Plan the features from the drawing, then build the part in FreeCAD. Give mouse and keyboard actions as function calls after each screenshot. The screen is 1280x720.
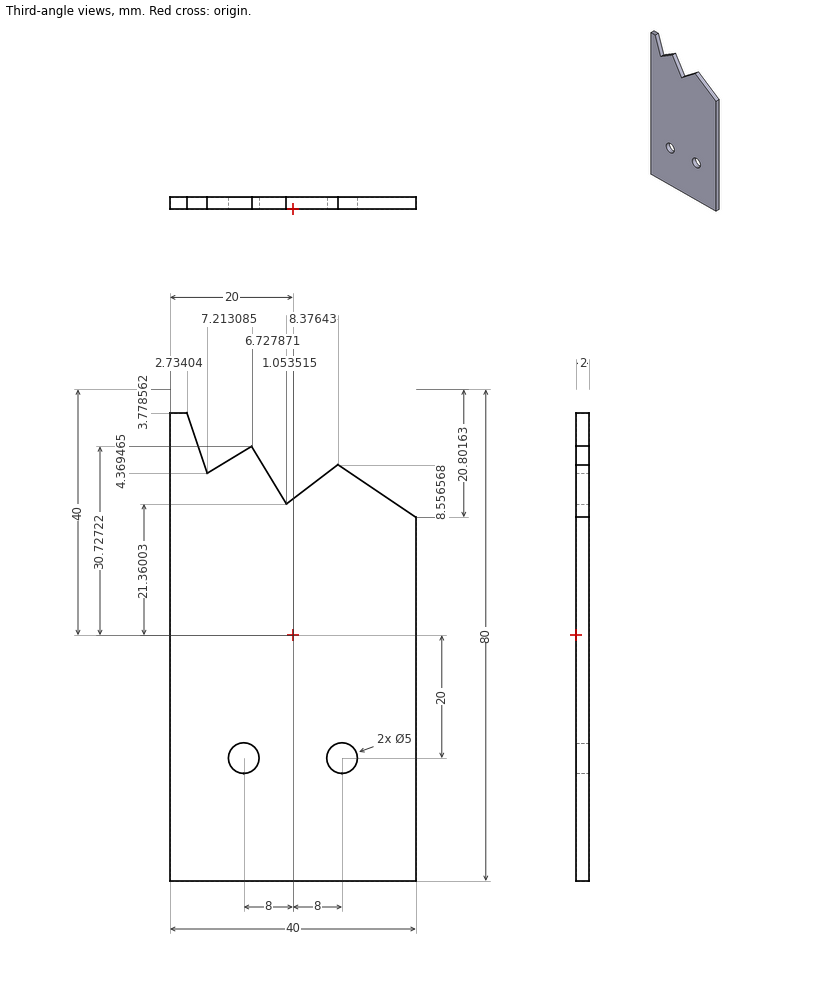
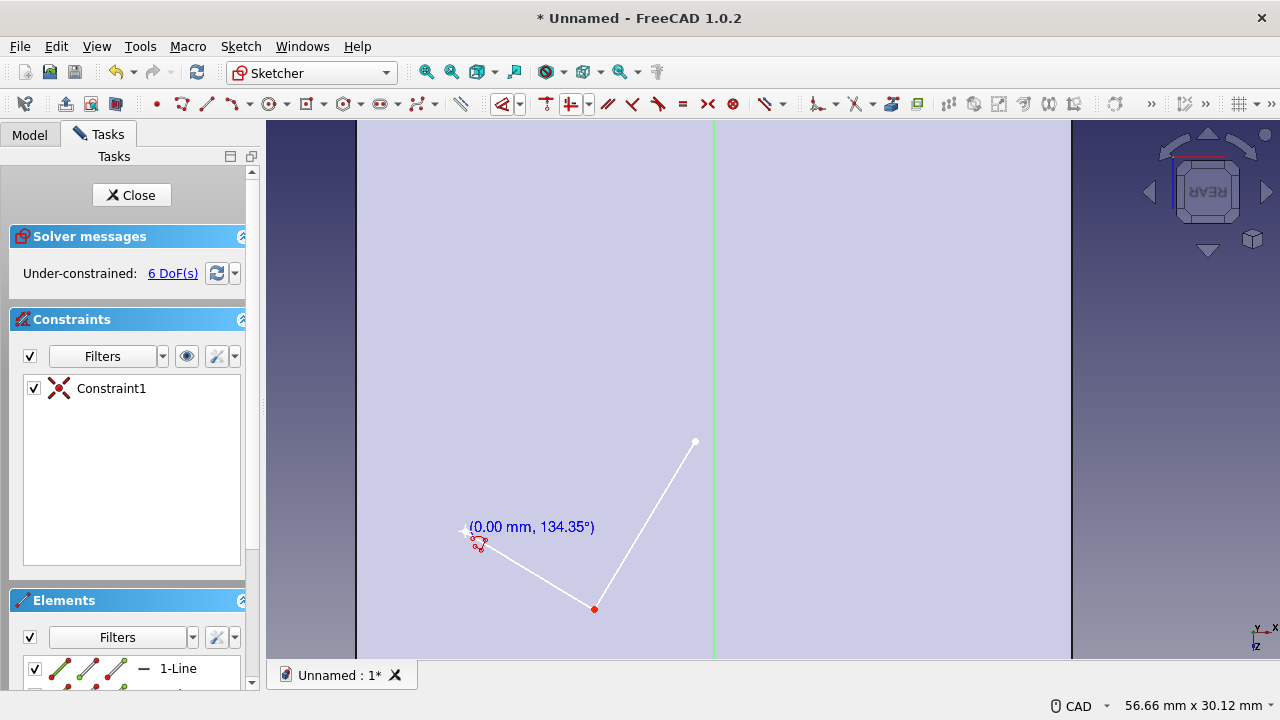
scroll(697, 367, down, 4)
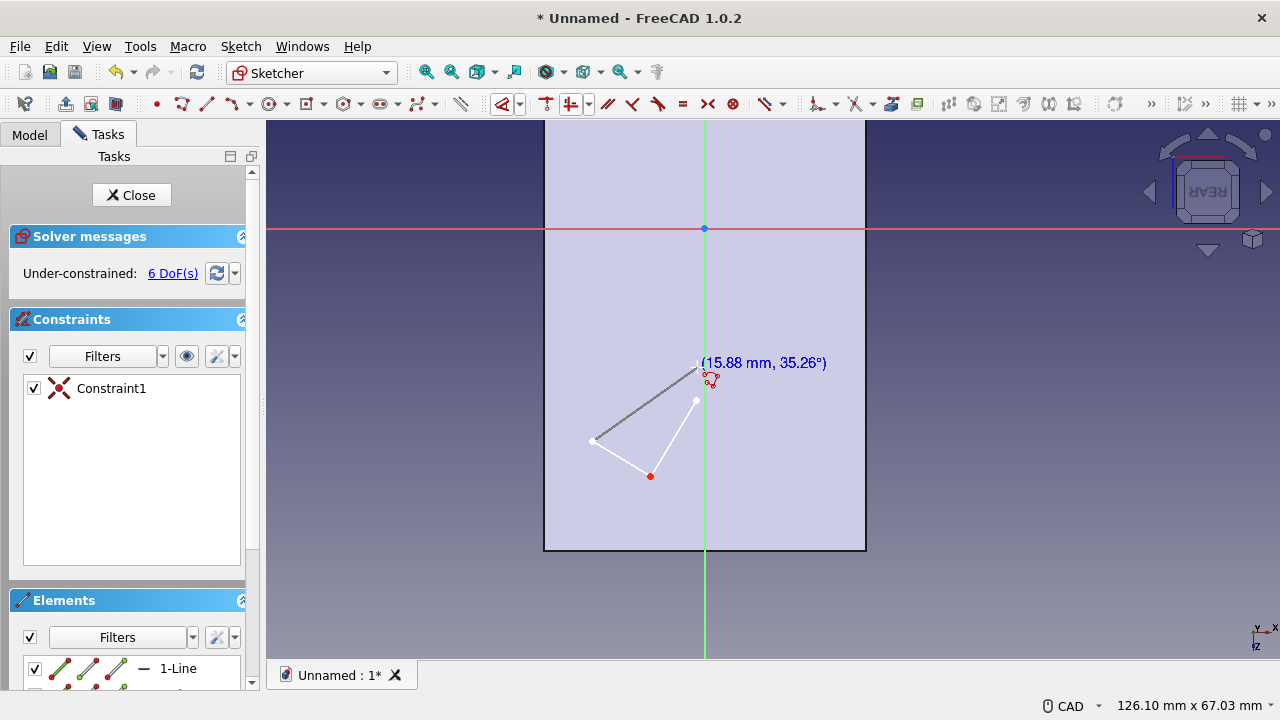
click(566, 520)
click(544, 520)
click(544, 551)
click(866, 551)
click(866, 383)
click(764, 452)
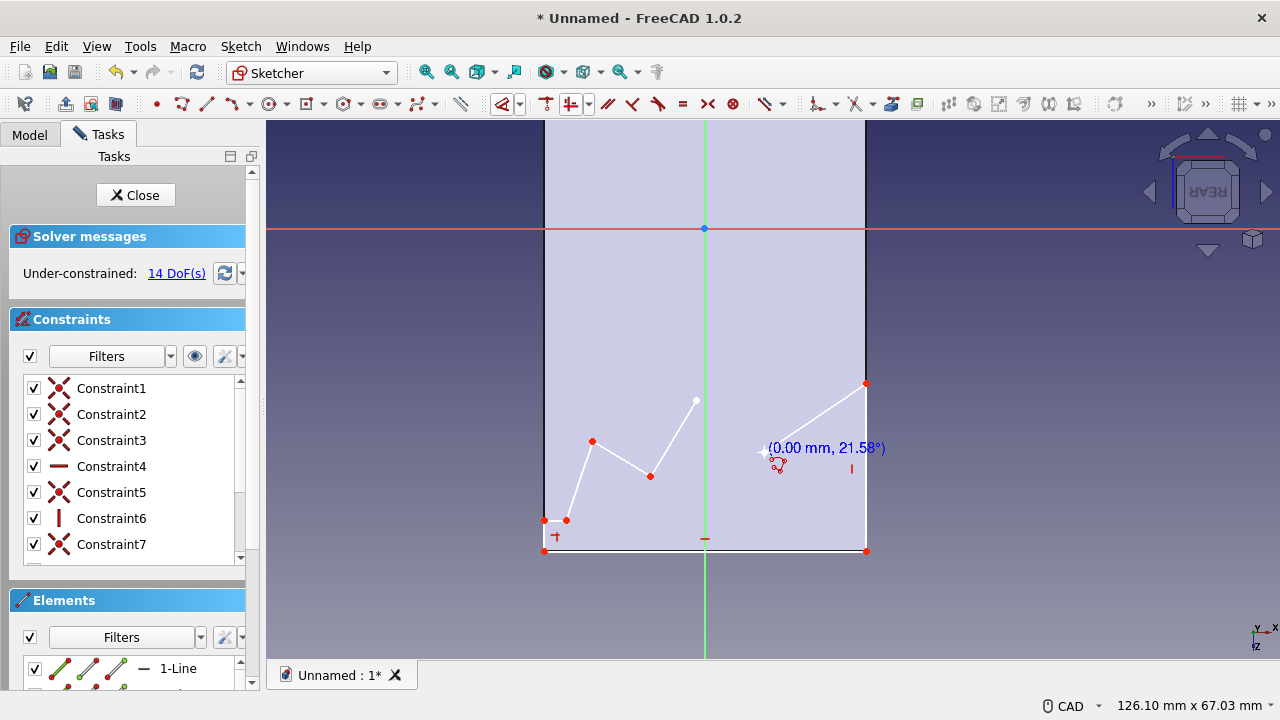
scroll(696, 401, up, 4)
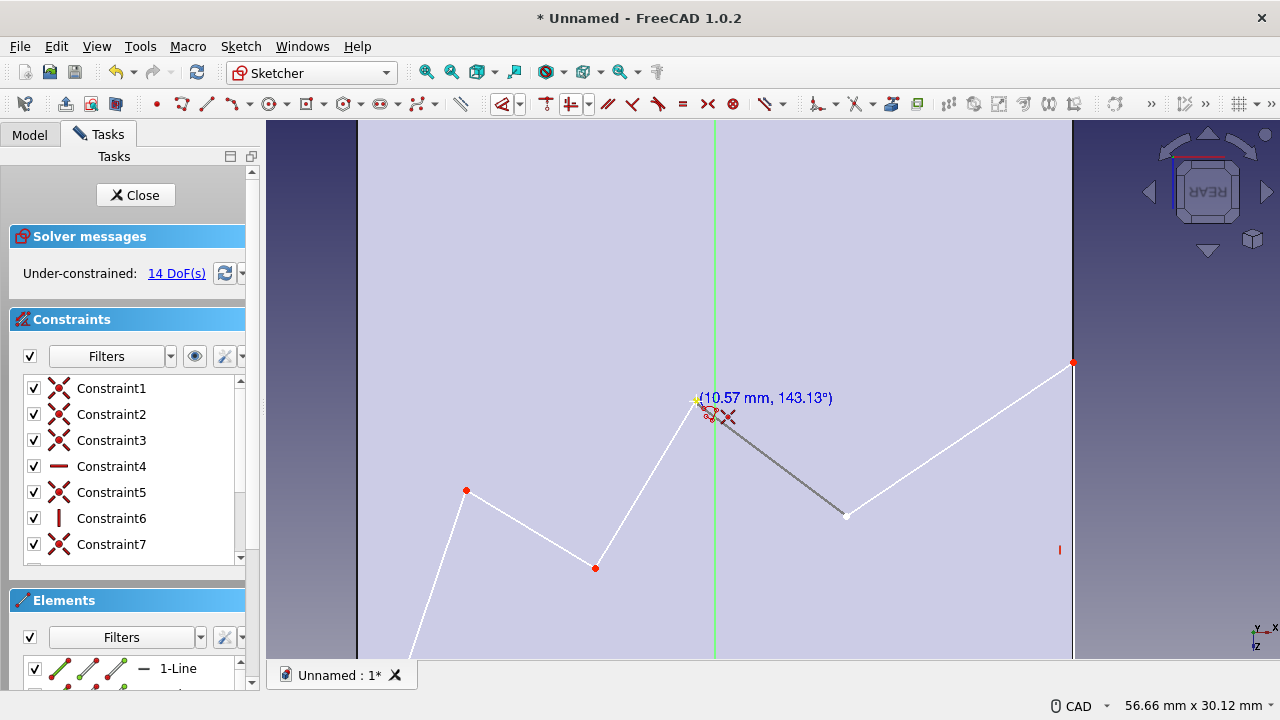
click(696, 400)
key(Escape)
key(Escape)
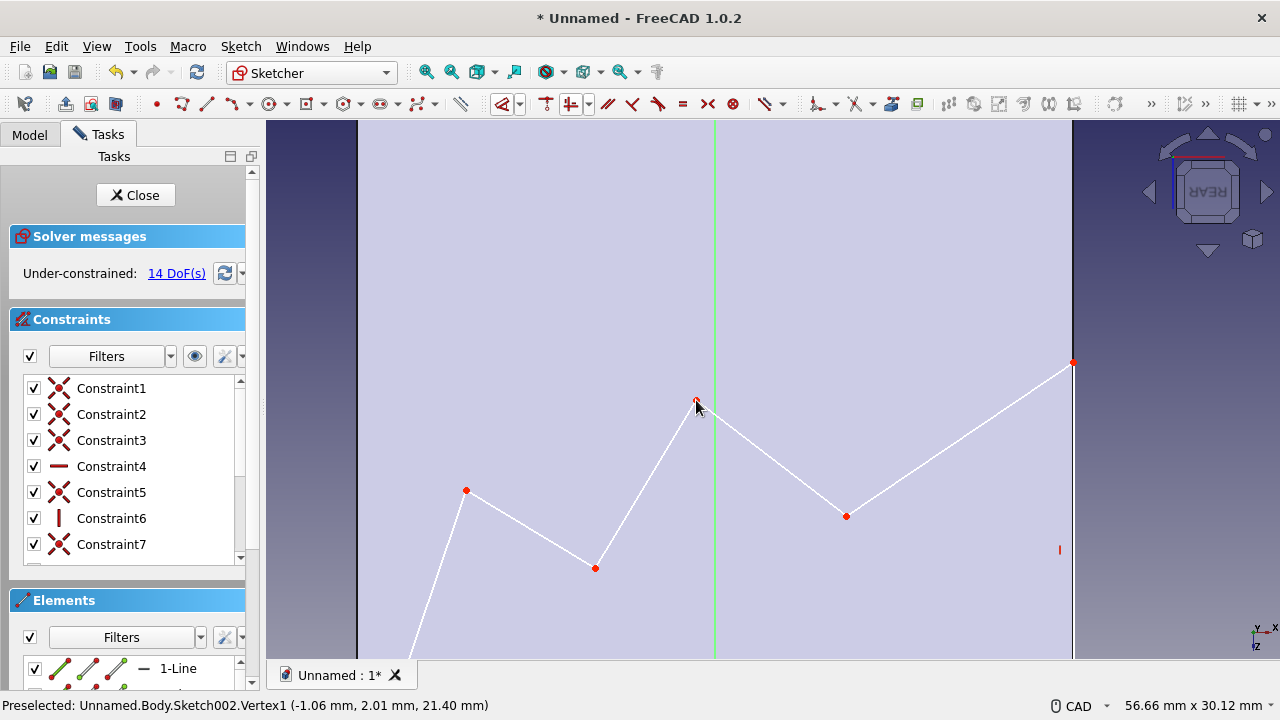
scroll(696, 401, down, 4)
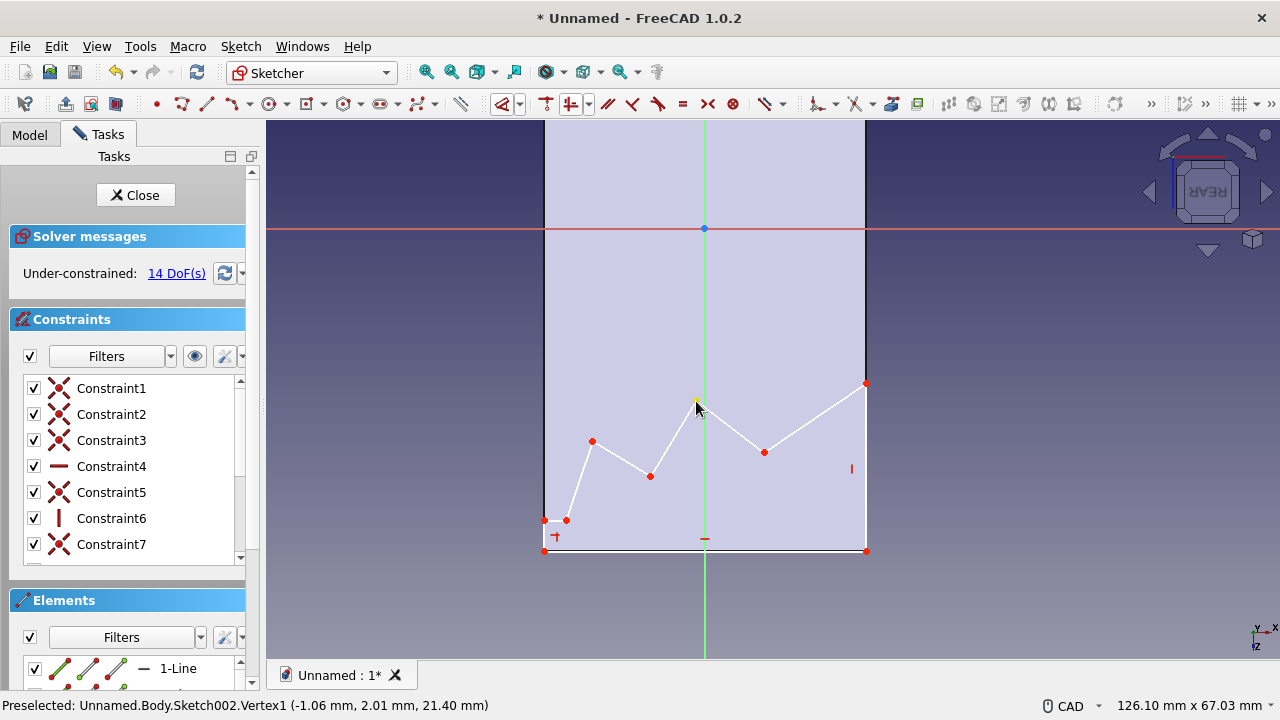
click(641, 552)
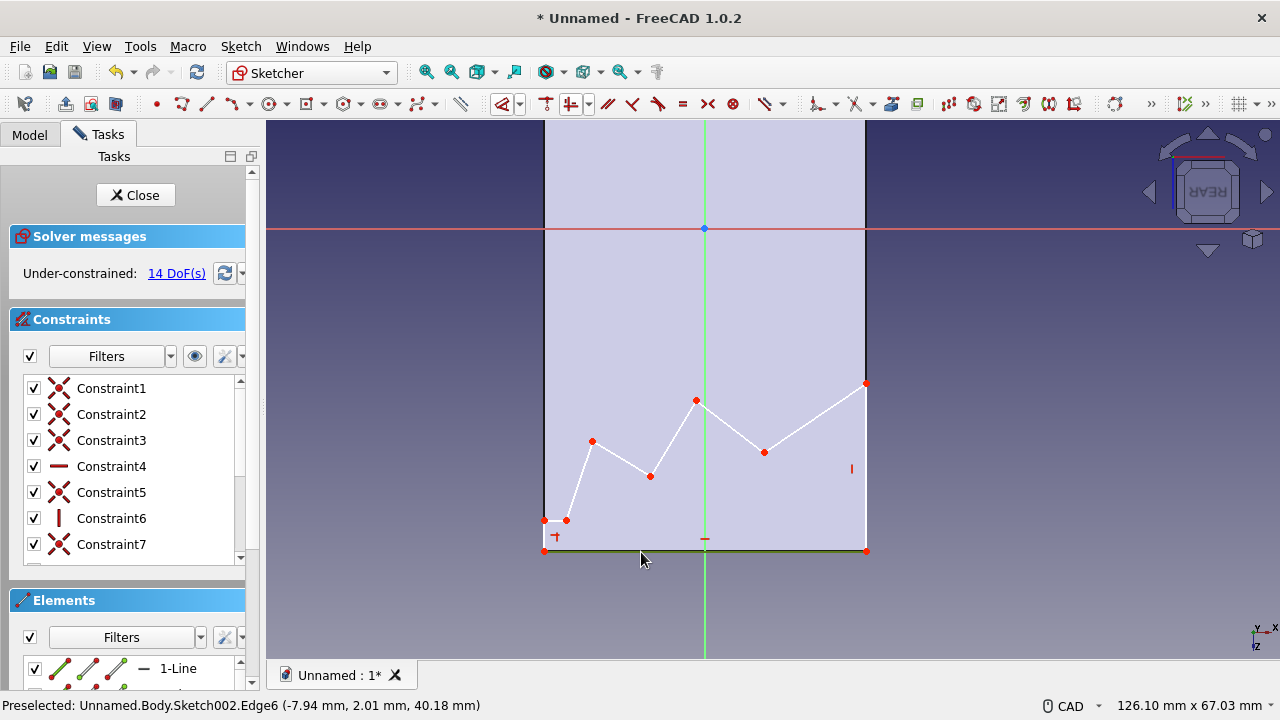
key(l)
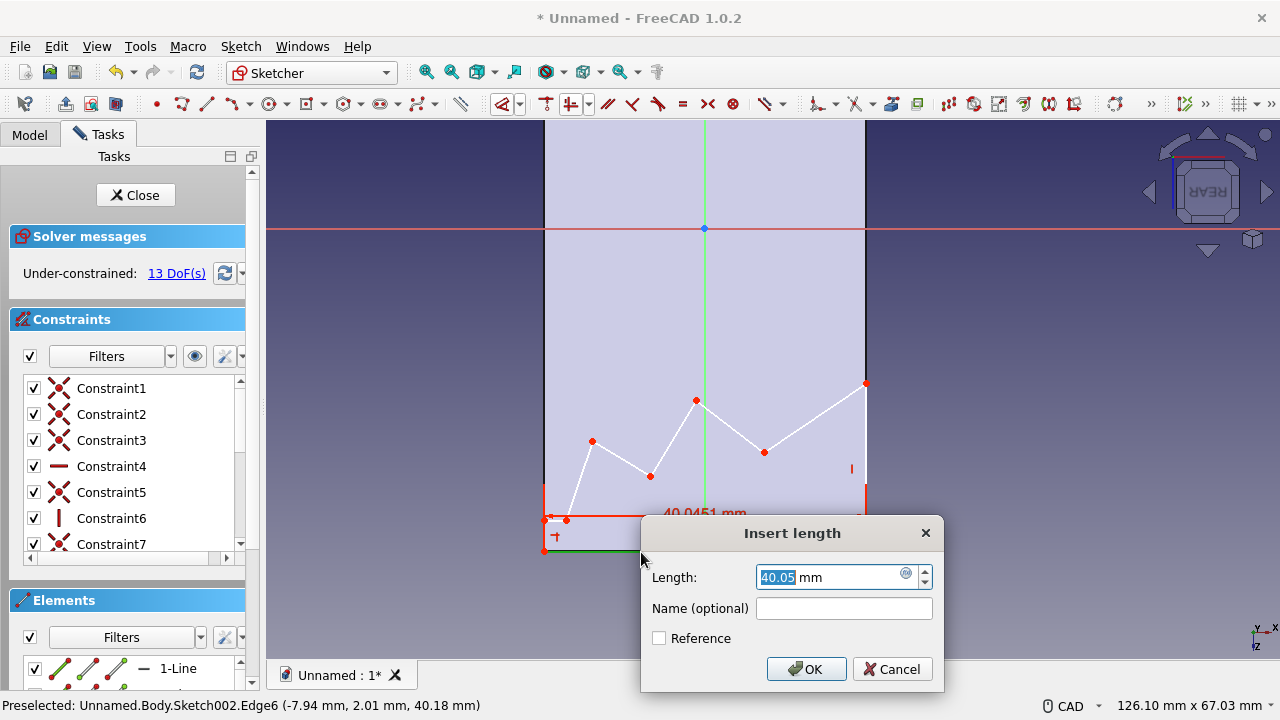
text(40)
key(Return)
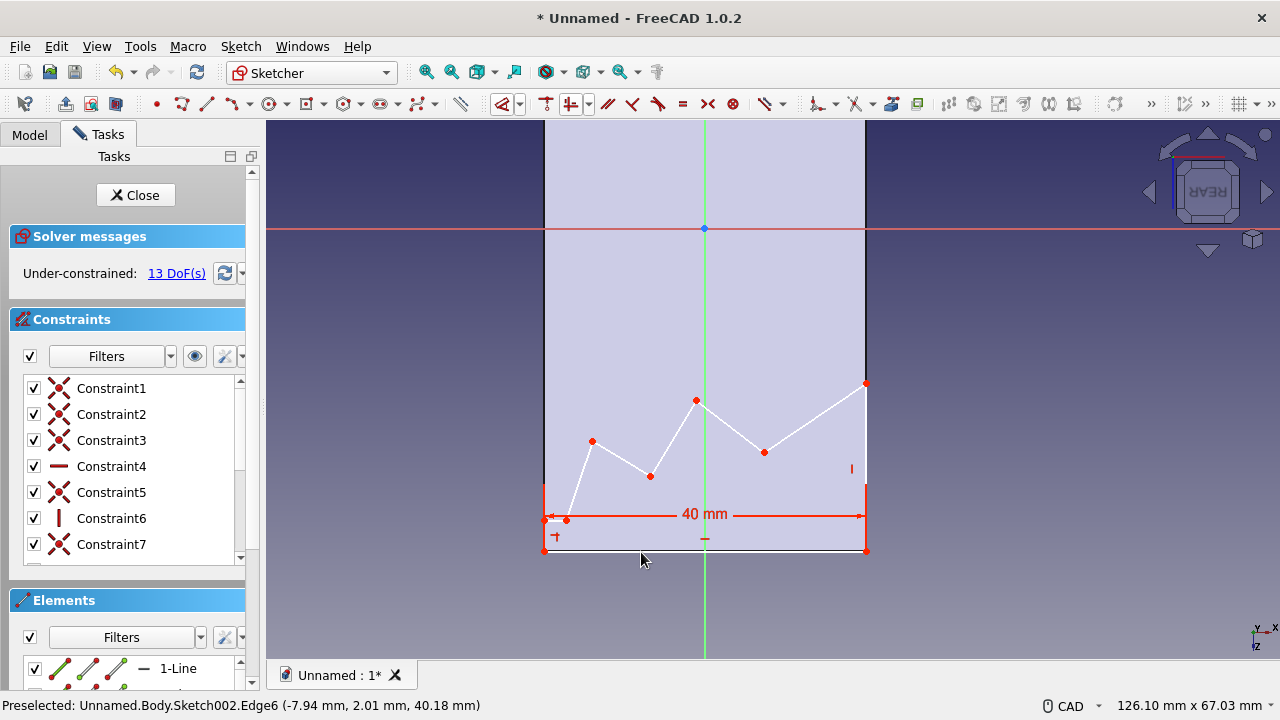
click(544, 521)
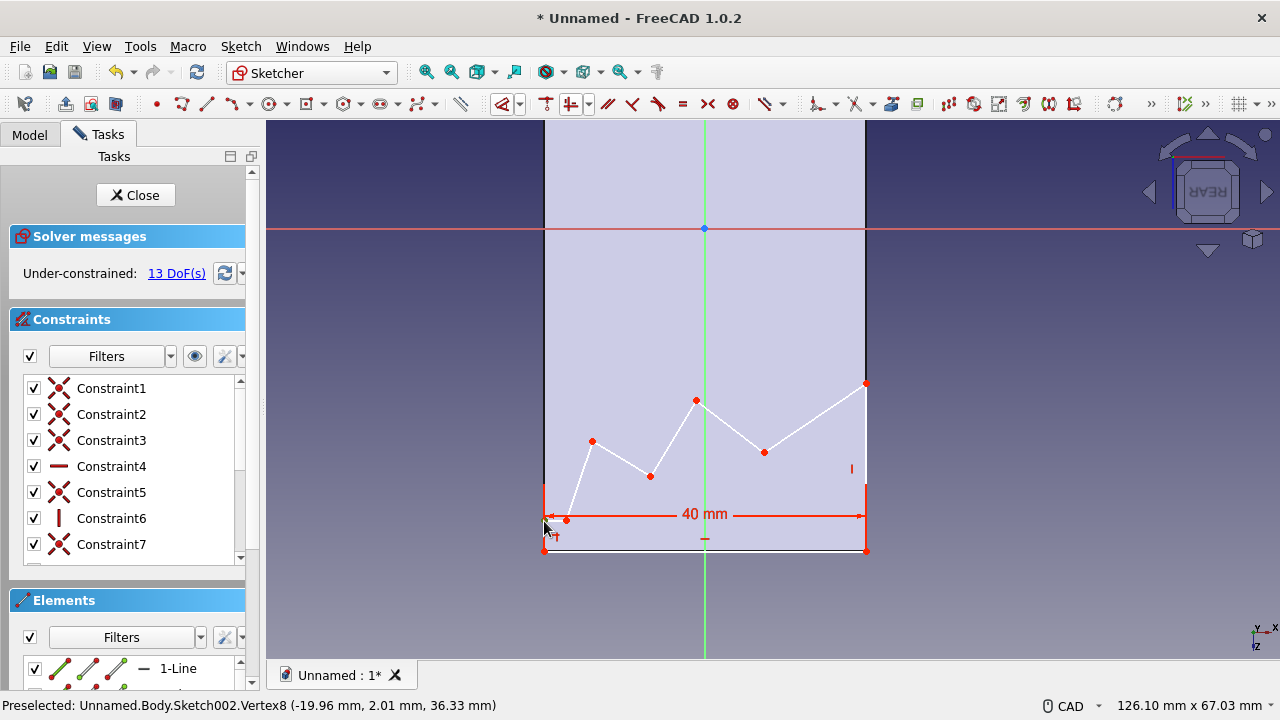
key(l)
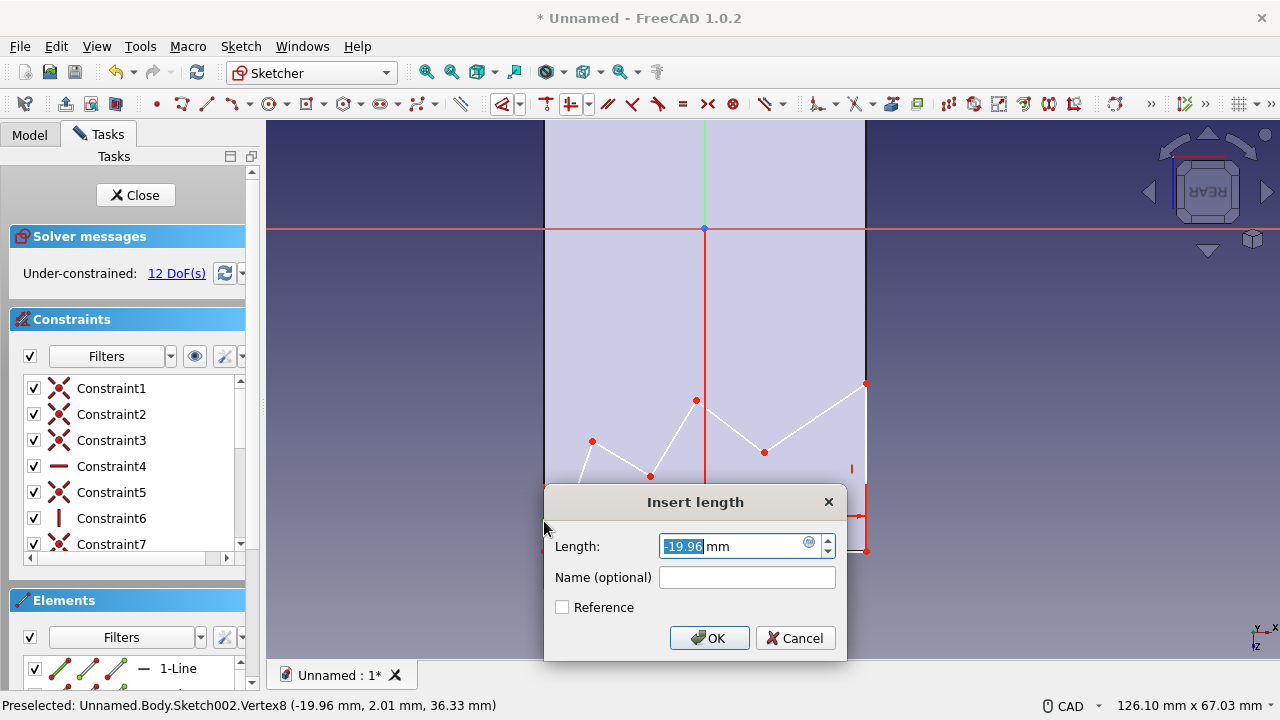
text(-20)
key(Return)